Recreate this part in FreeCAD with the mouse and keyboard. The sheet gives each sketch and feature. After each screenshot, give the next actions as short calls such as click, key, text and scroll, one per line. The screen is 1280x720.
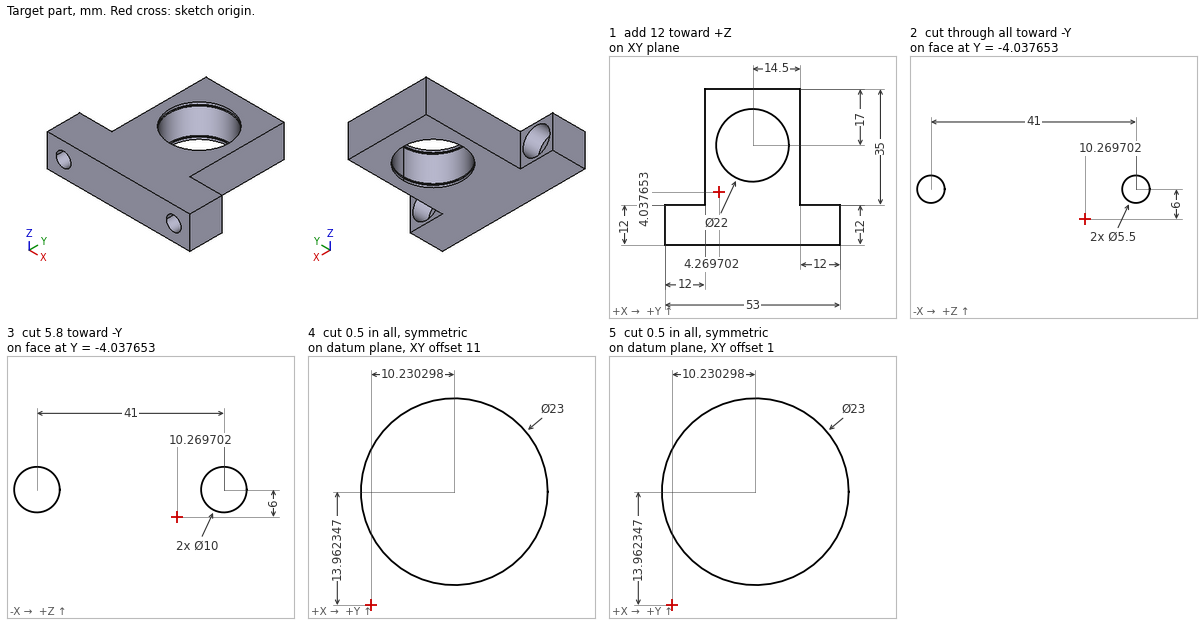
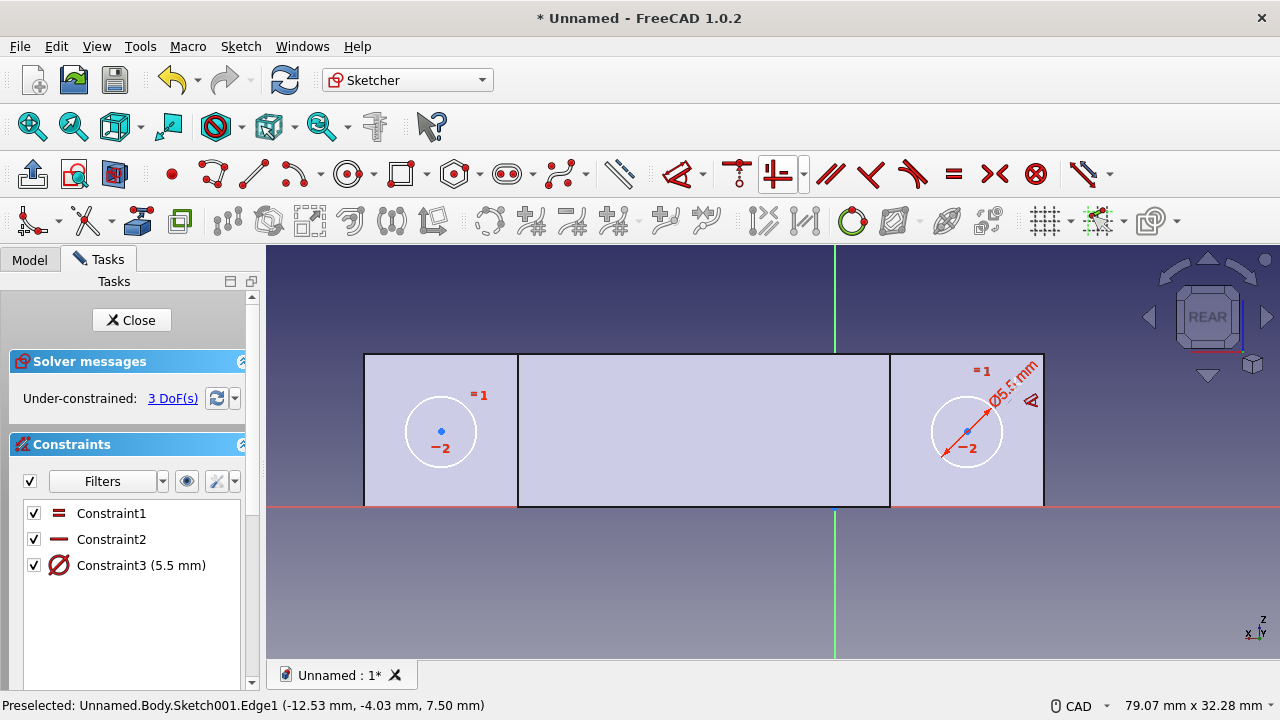
click(967, 432)
click(1001, 470)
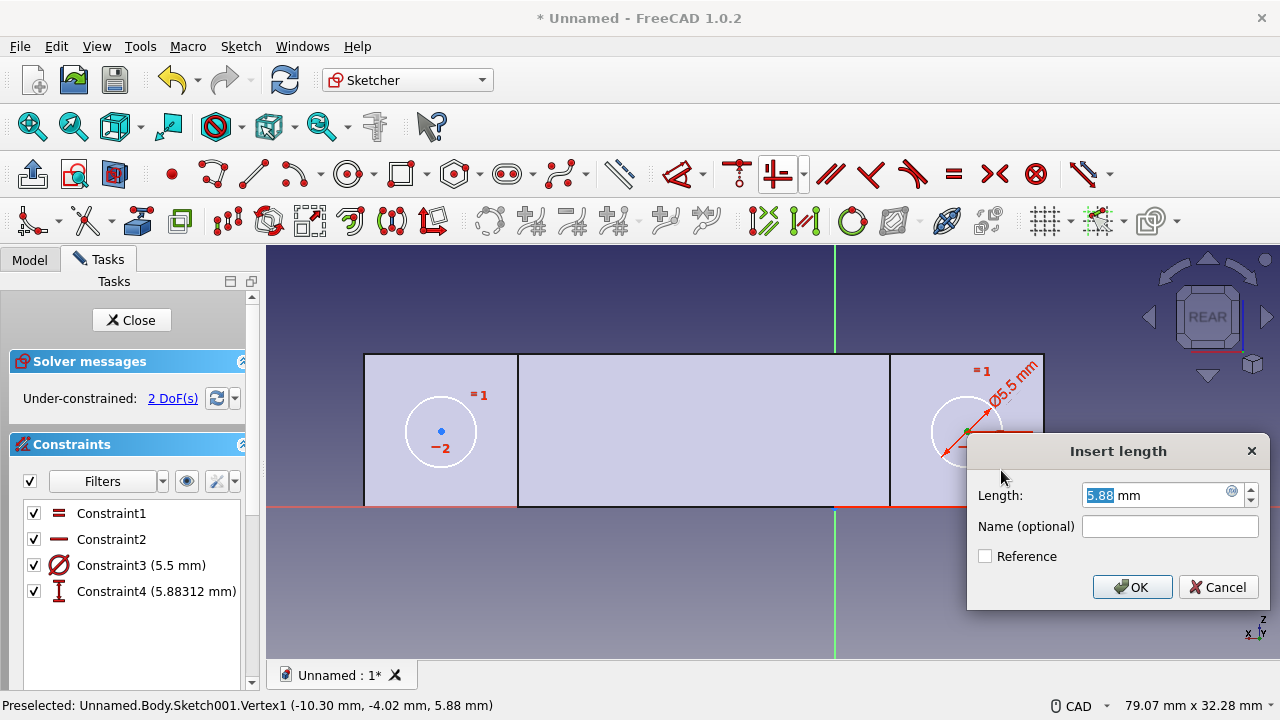
text(6)
key(Return)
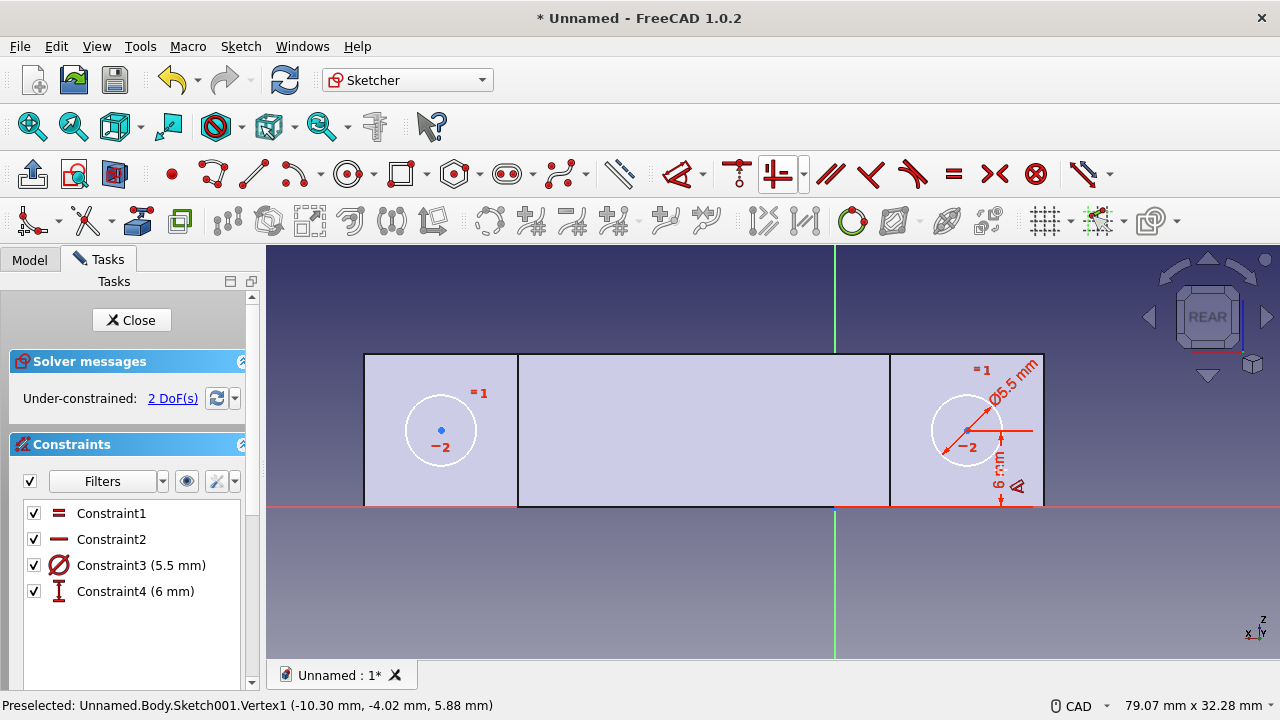
click(967, 431)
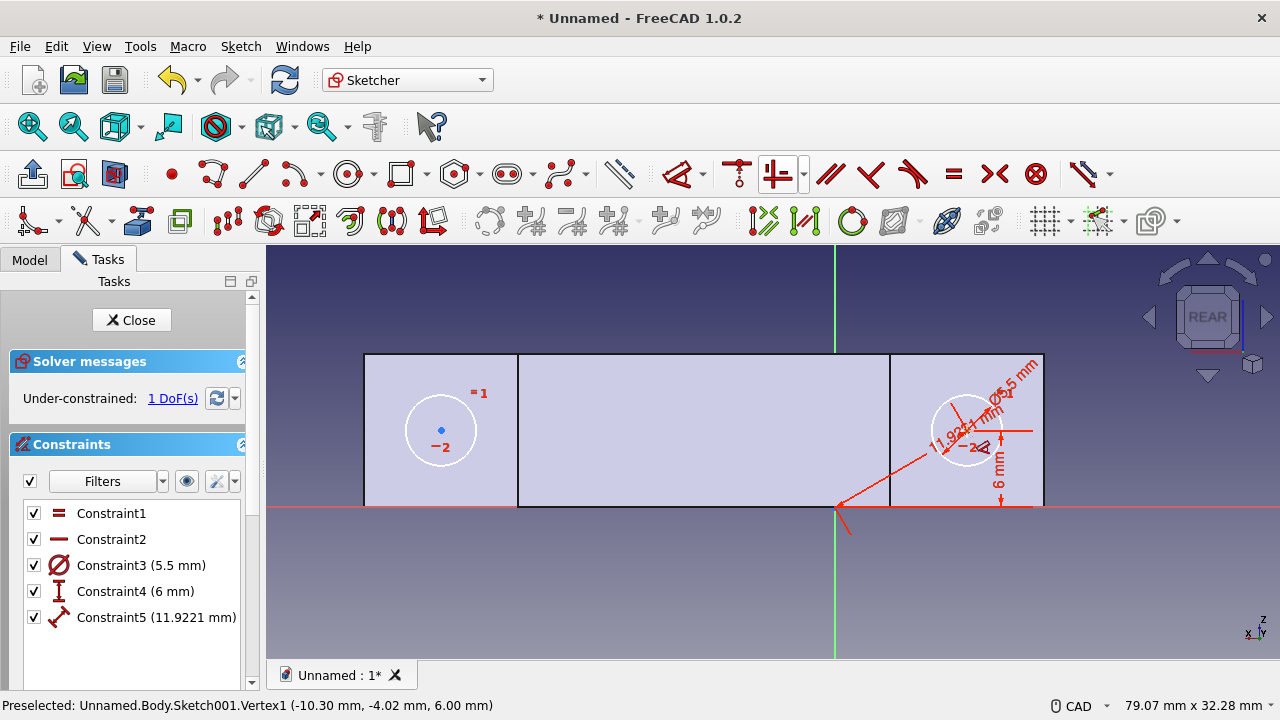
click(441, 431)
click(704, 397)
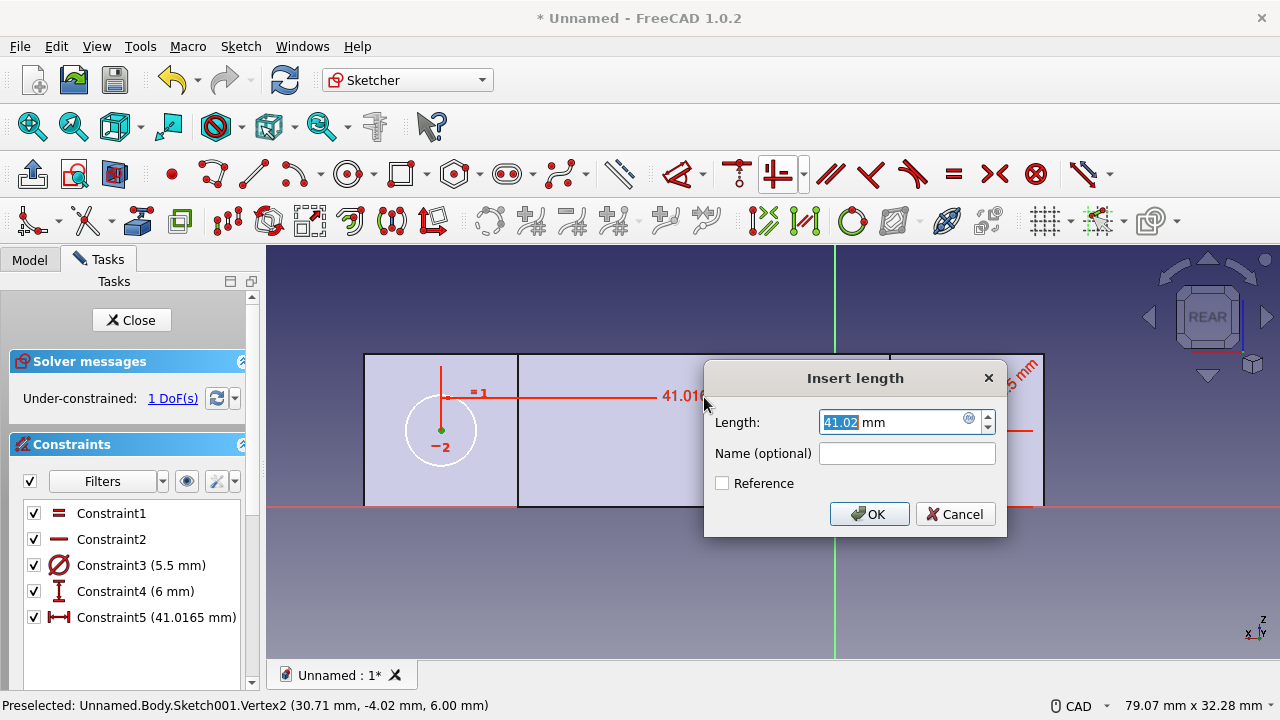
text(41)
key(Return)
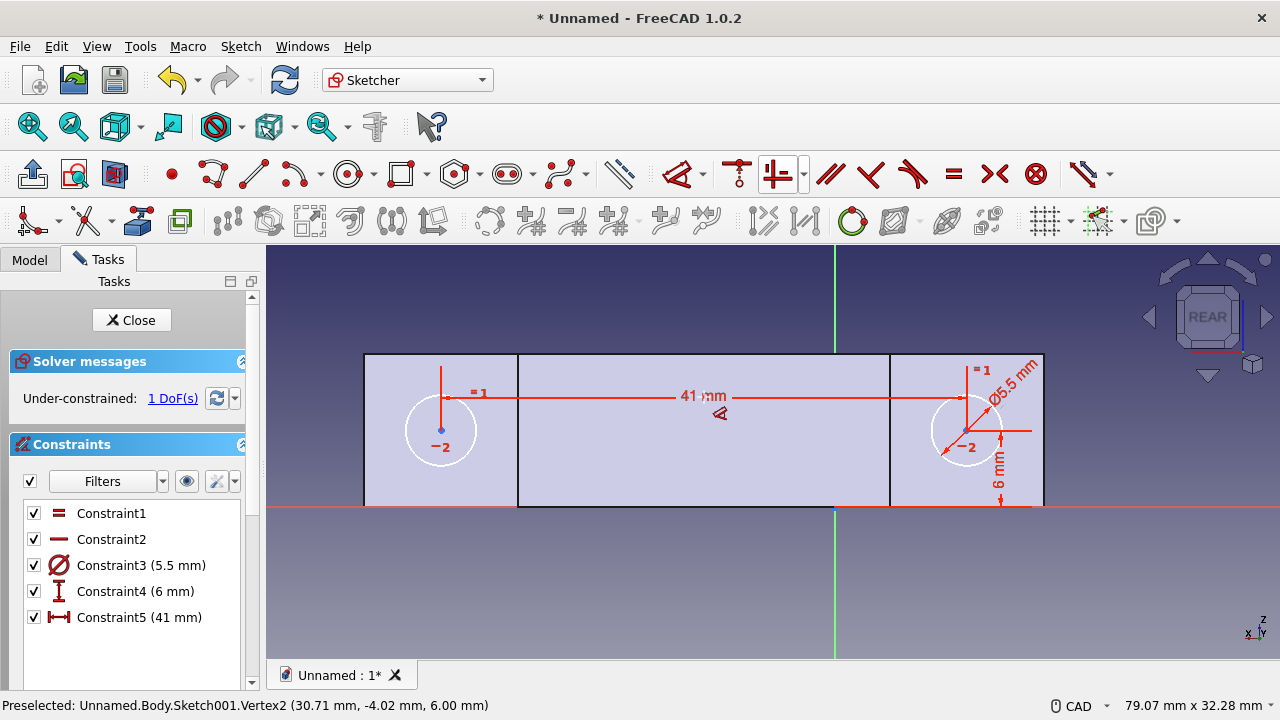
click(967, 431)
click(901, 541)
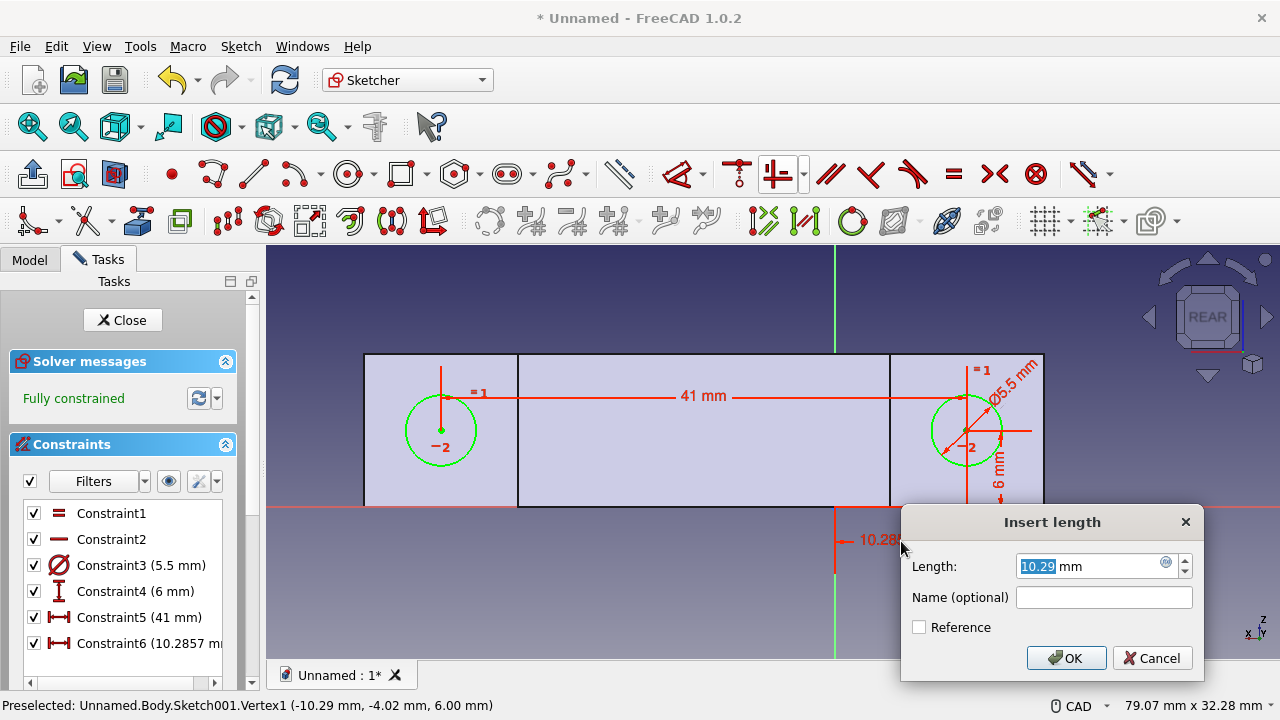
text(10.269702)
key(Return)
key(Escape)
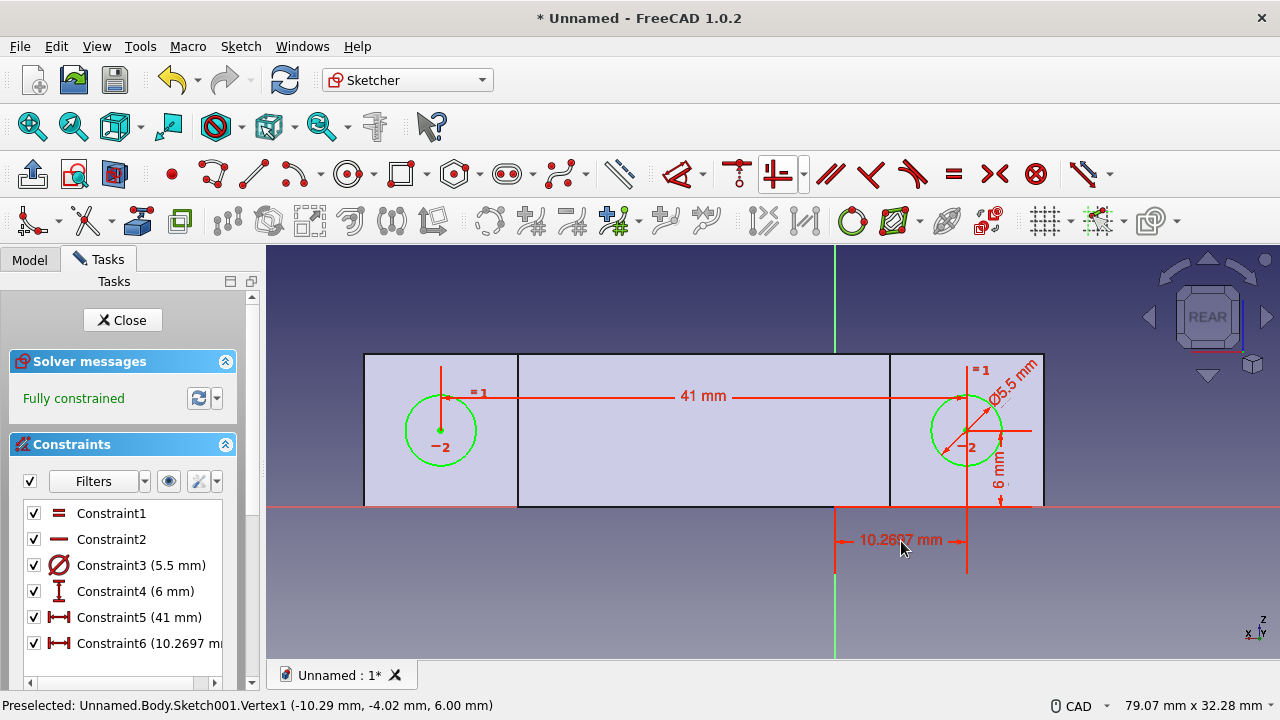
click(123, 320)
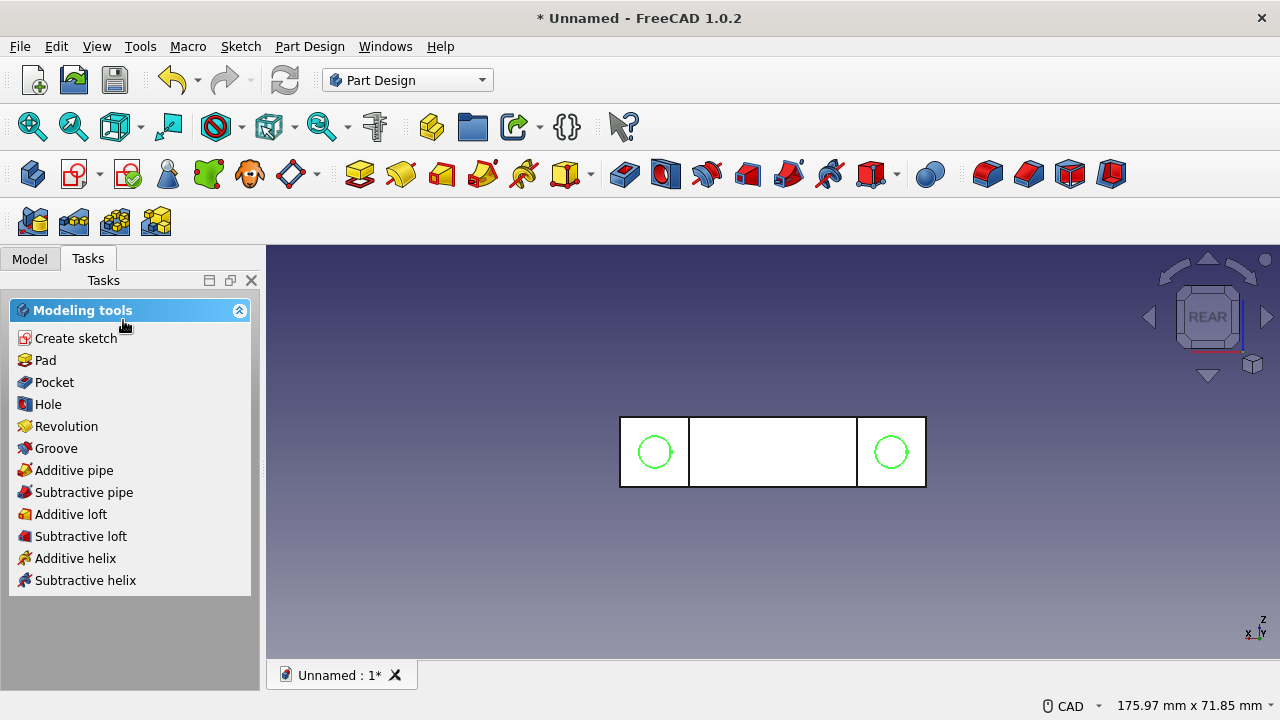
click(625, 174)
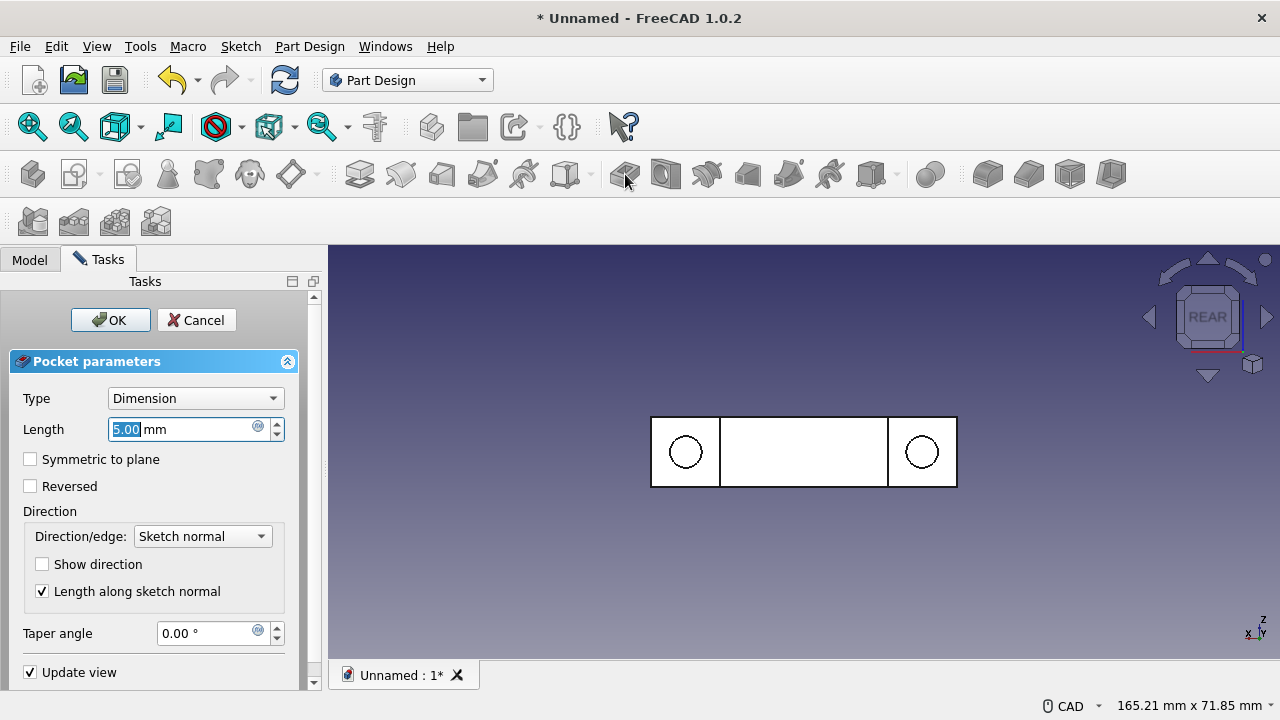
click(196, 398)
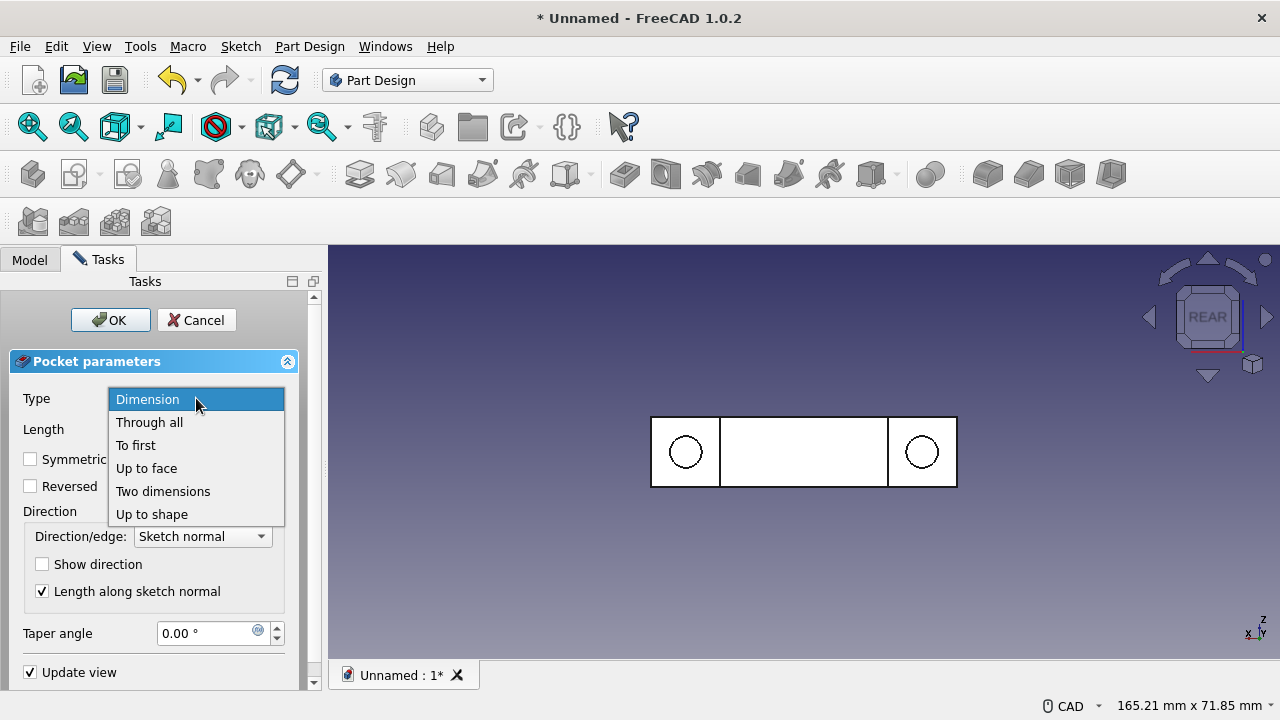
click(194, 422)